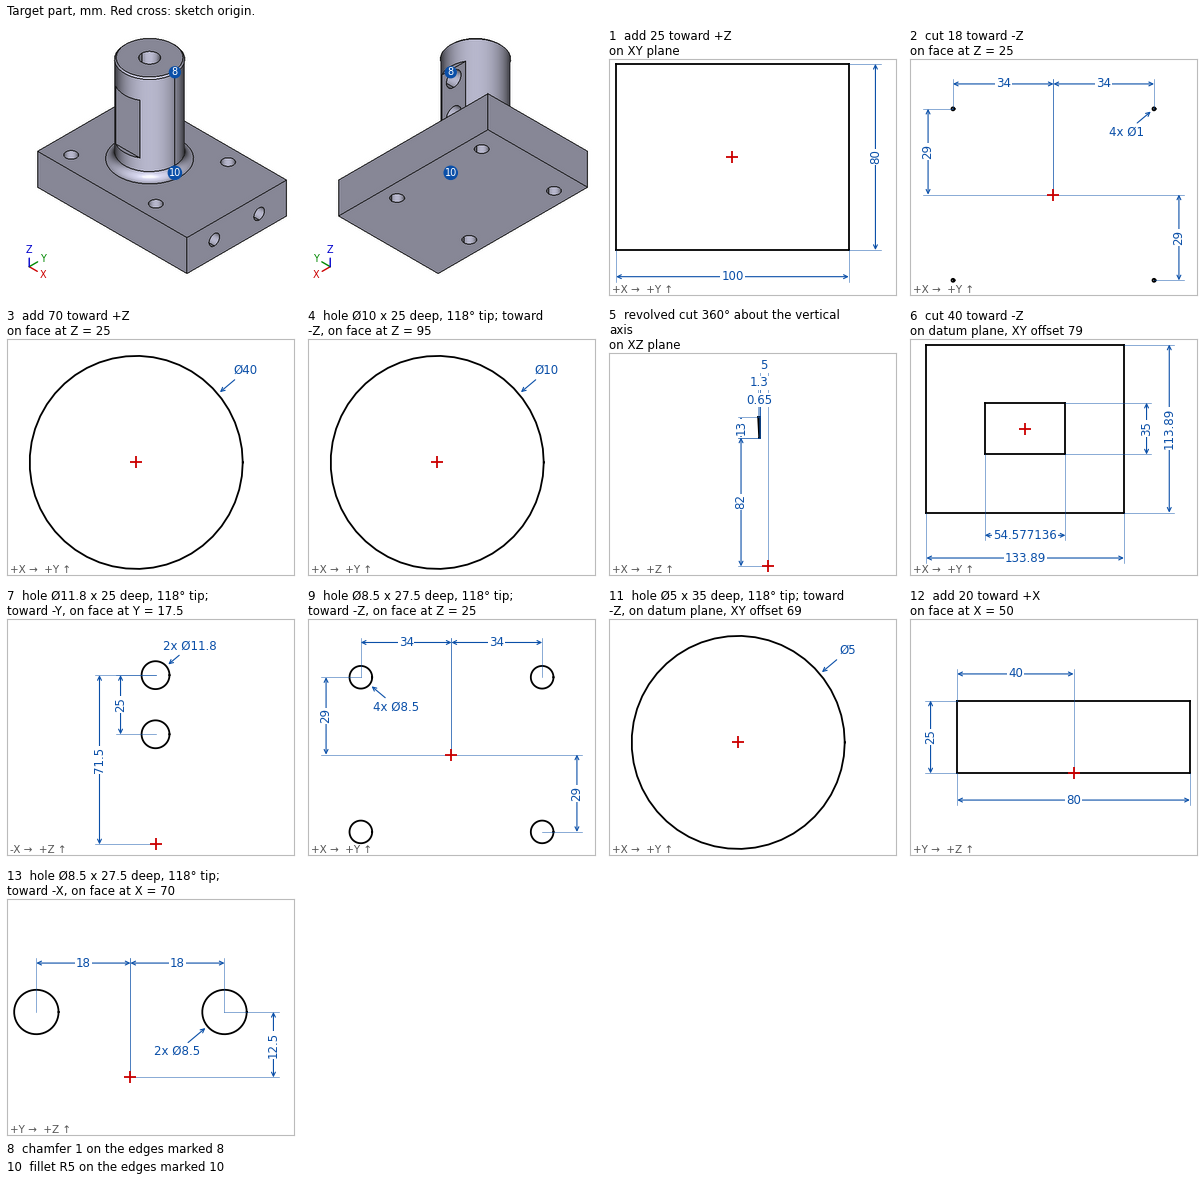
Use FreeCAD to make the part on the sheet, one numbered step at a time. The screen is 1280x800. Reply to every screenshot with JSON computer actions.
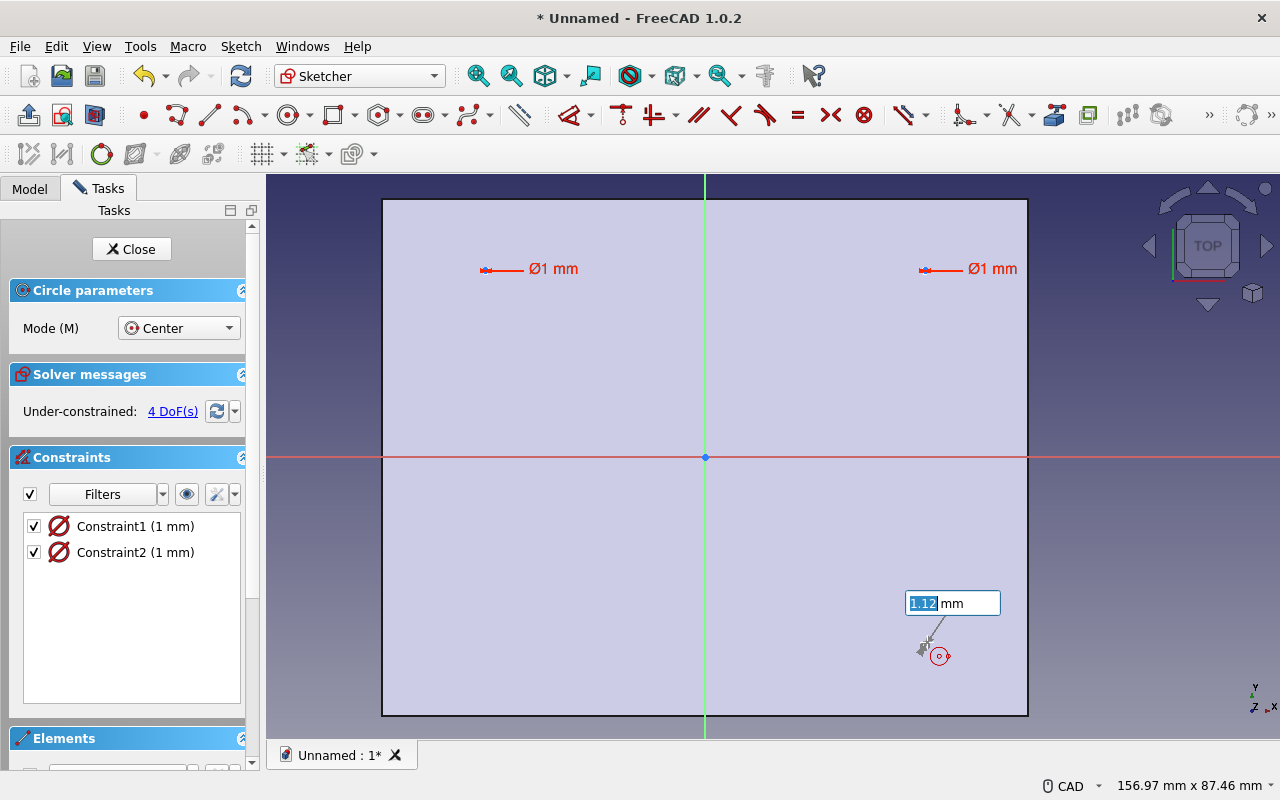
{"action": "type", "text": "1"}
{"action": "key", "text": "Return"}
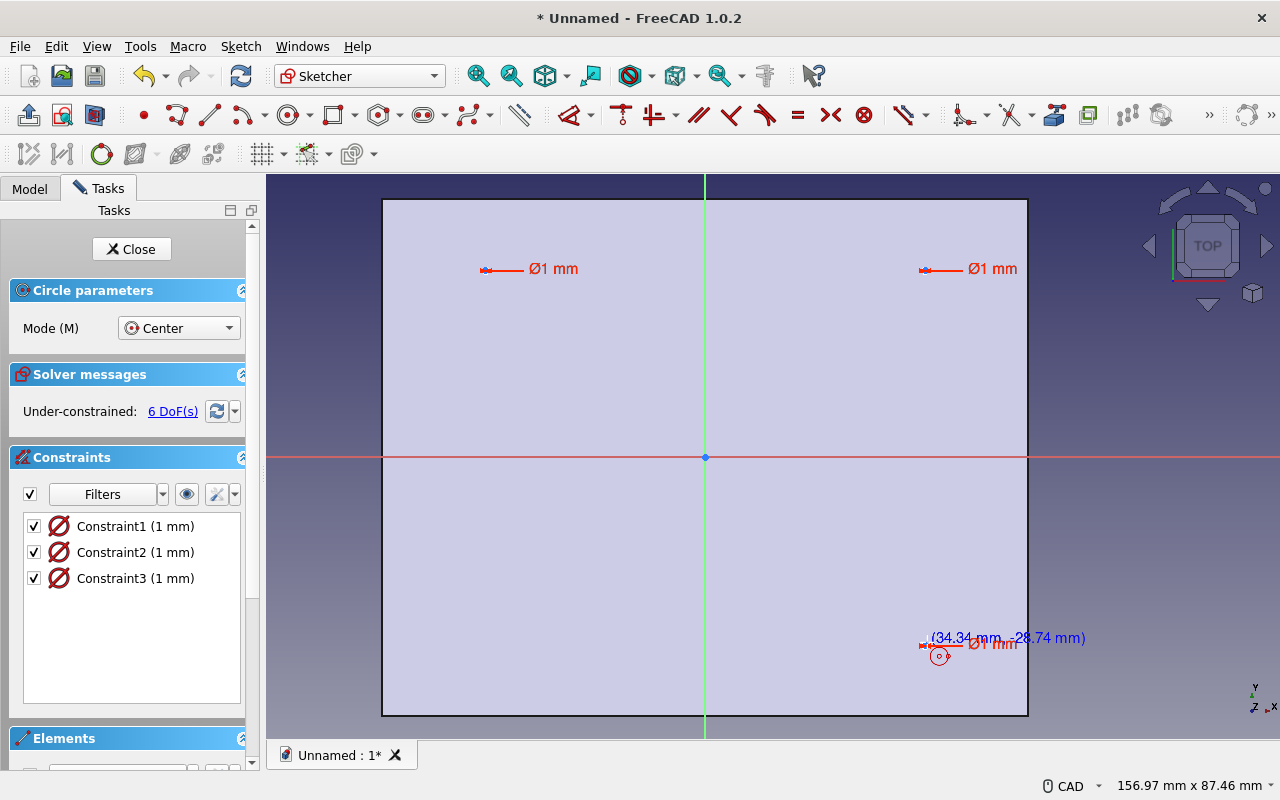
{"action": "scroll", "coordinate": [486, 645], "scroll_direction": "up", "scroll_amount": 10}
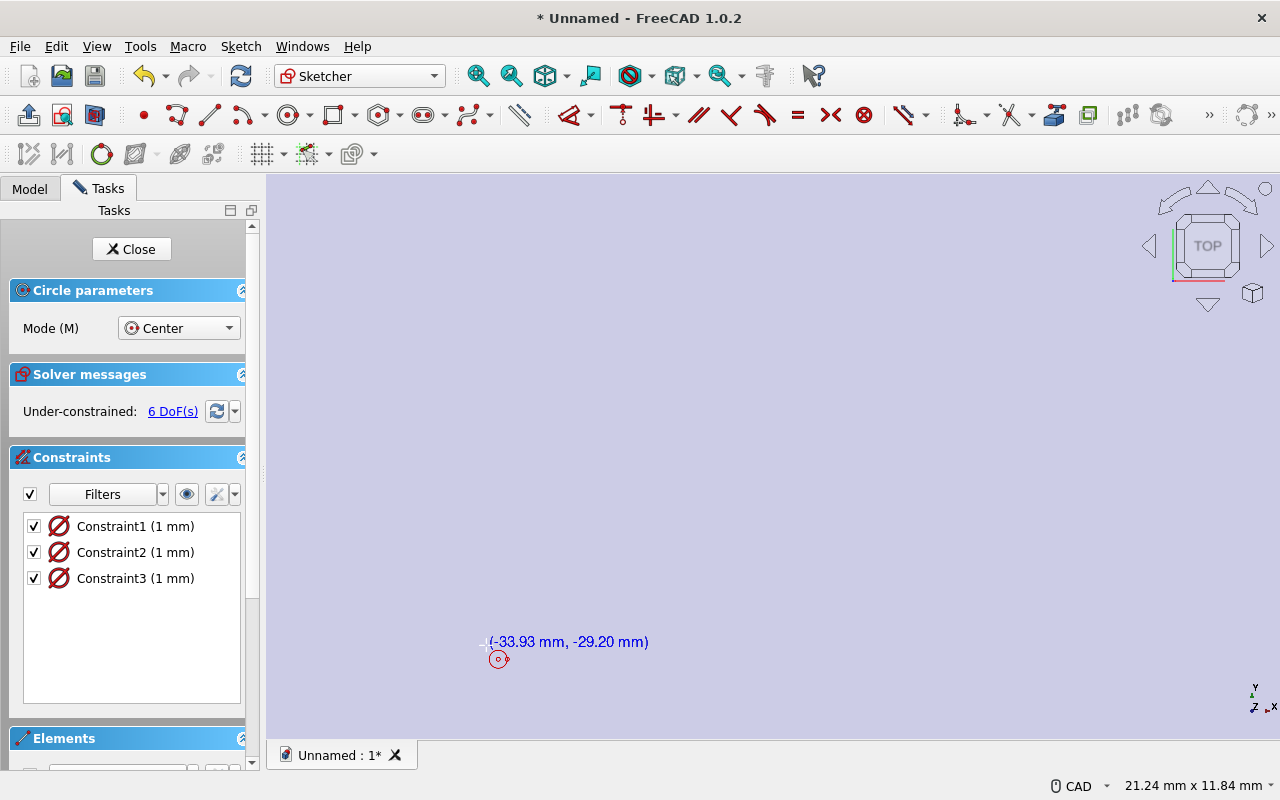
{"action": "scroll", "coordinate": [485, 645], "scroll_direction": "down", "scroll_amount": 10}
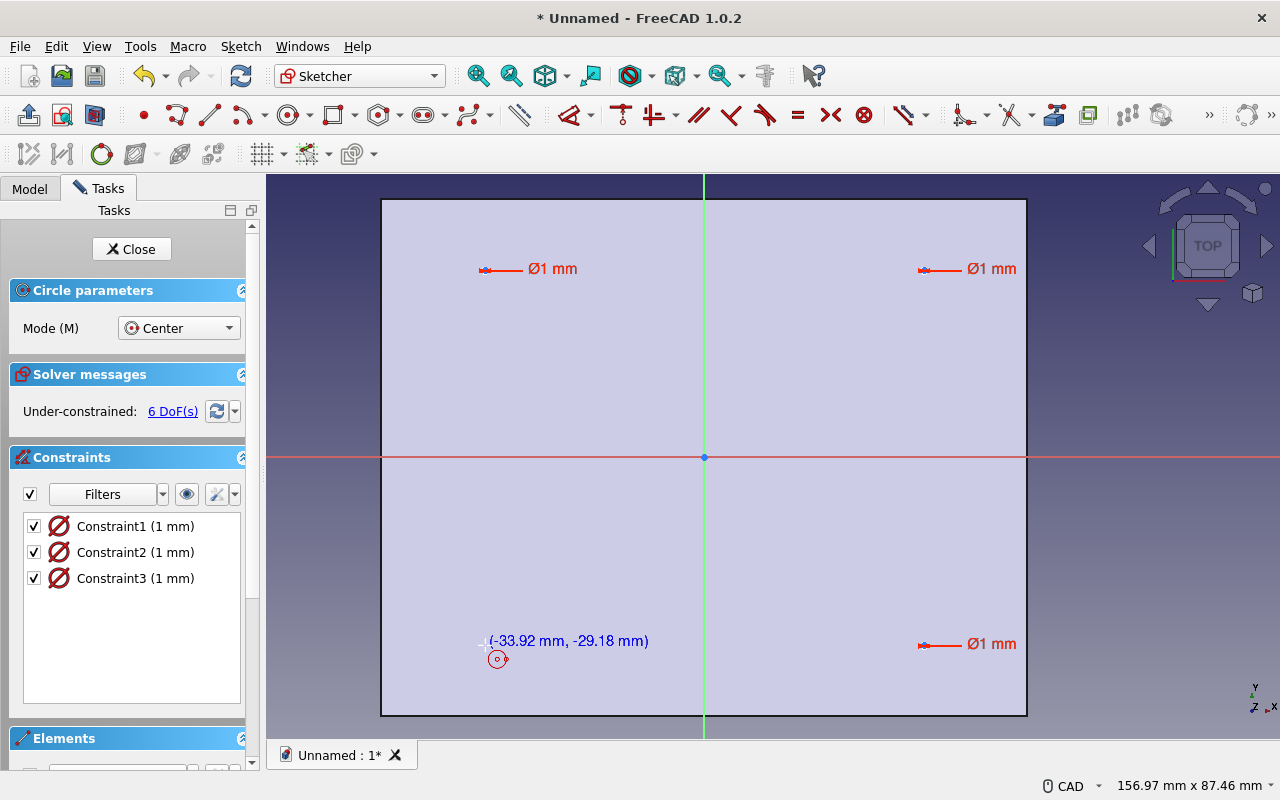
{"action": "left_click", "coordinate": [485, 645]}
{"action": "mouse_move", "coordinate": [487, 642]}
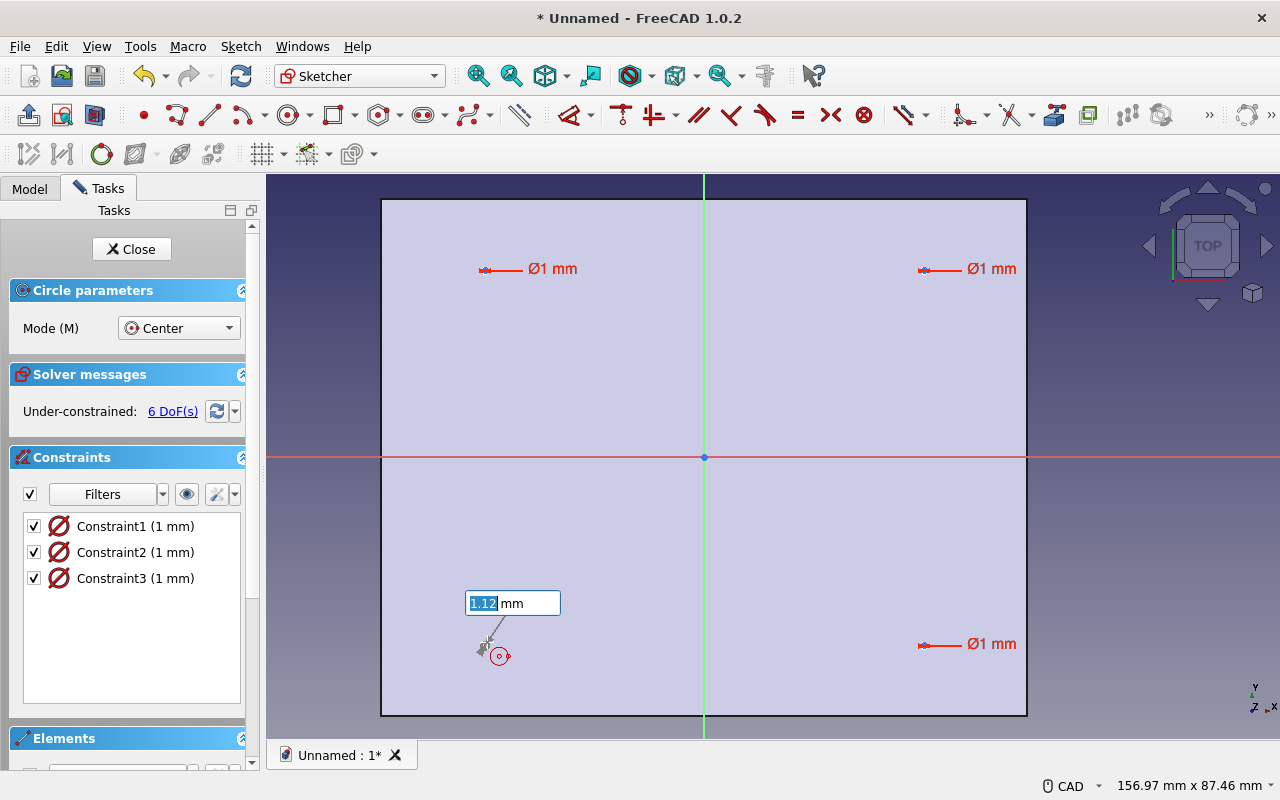
{"action": "type", "text": "1"}
{"action": "key", "text": "Return"}
{"action": "key", "text": "Escape"}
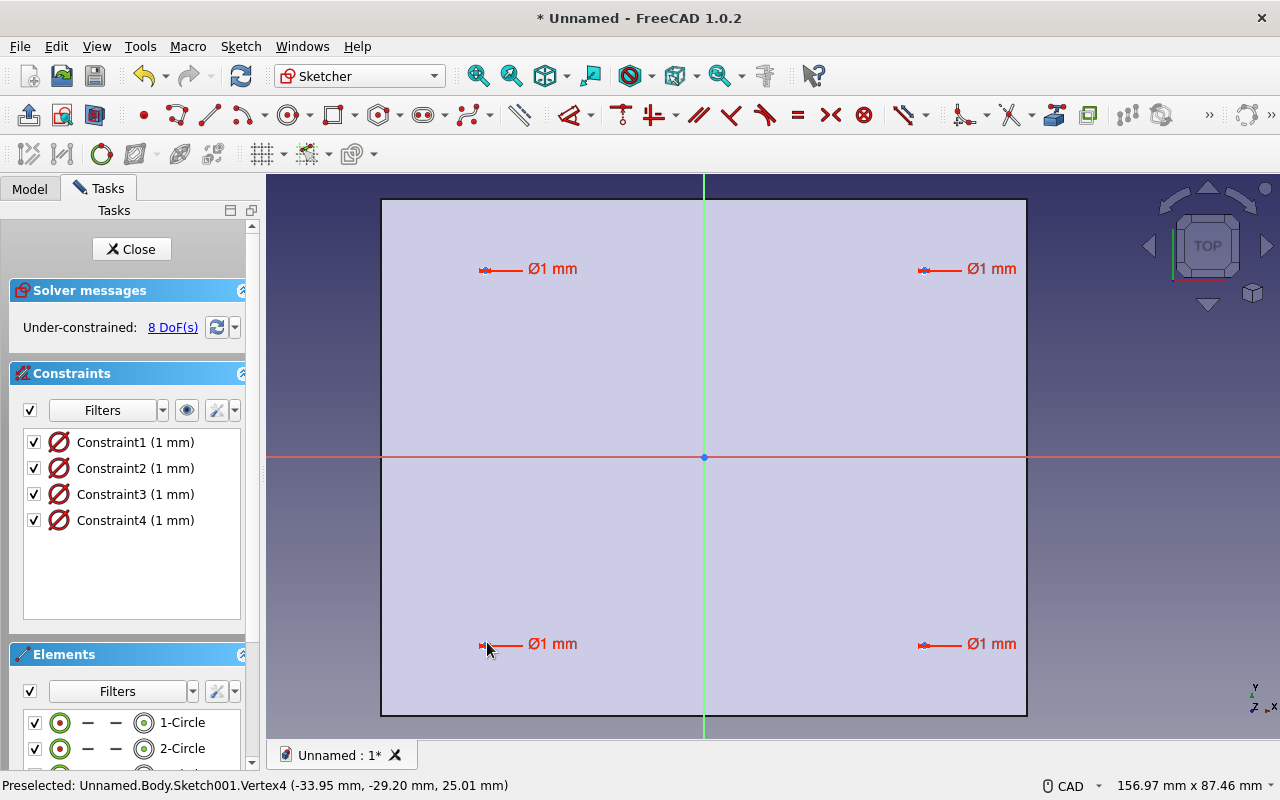
{"action": "left_click", "coordinate": [485, 271]}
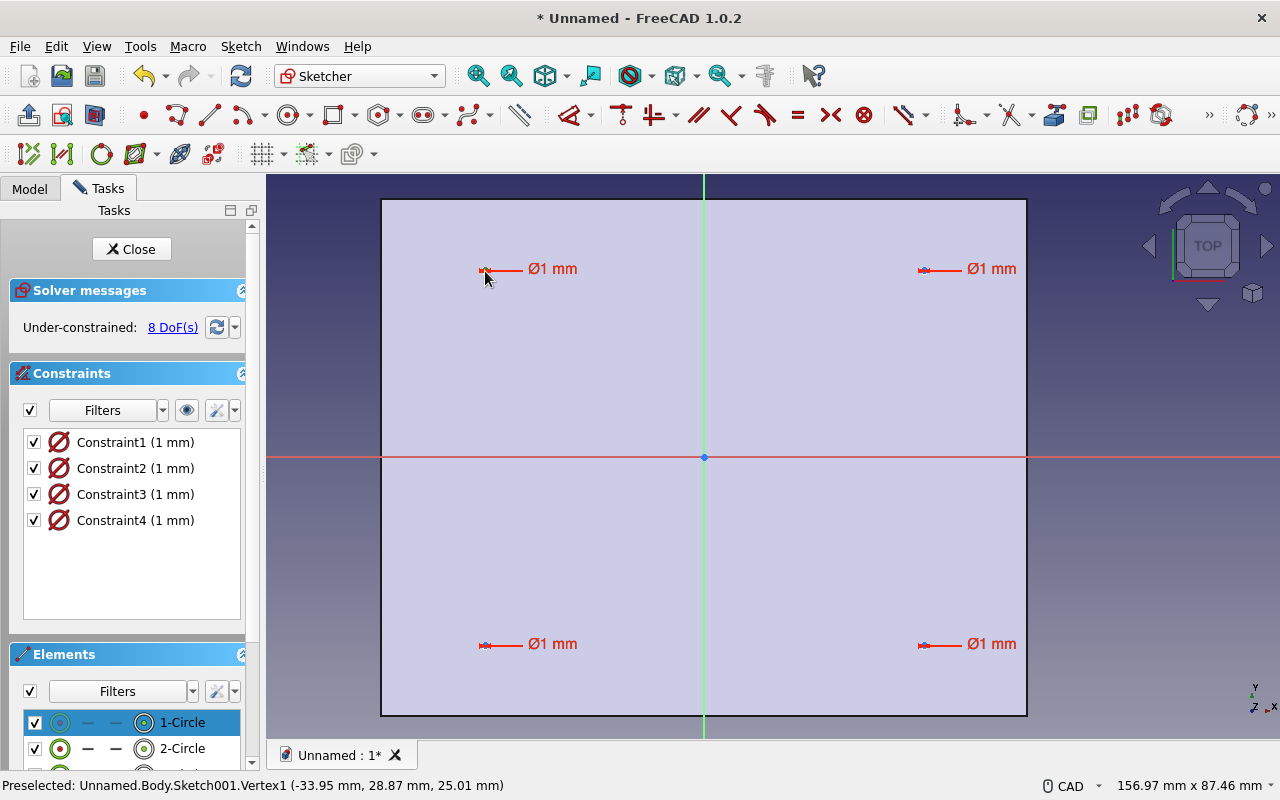
{"action": "left_click", "coordinate": [924, 271]}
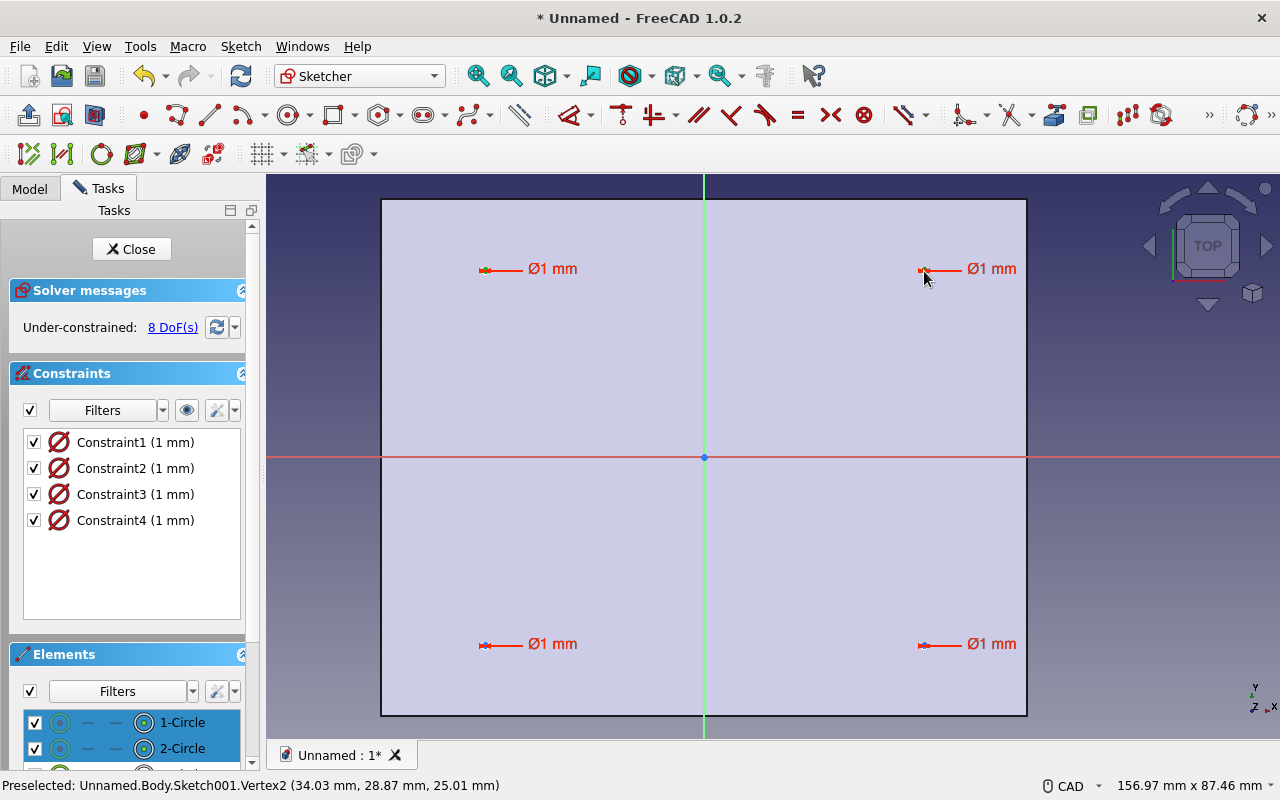
{"action": "key", "text": "h"}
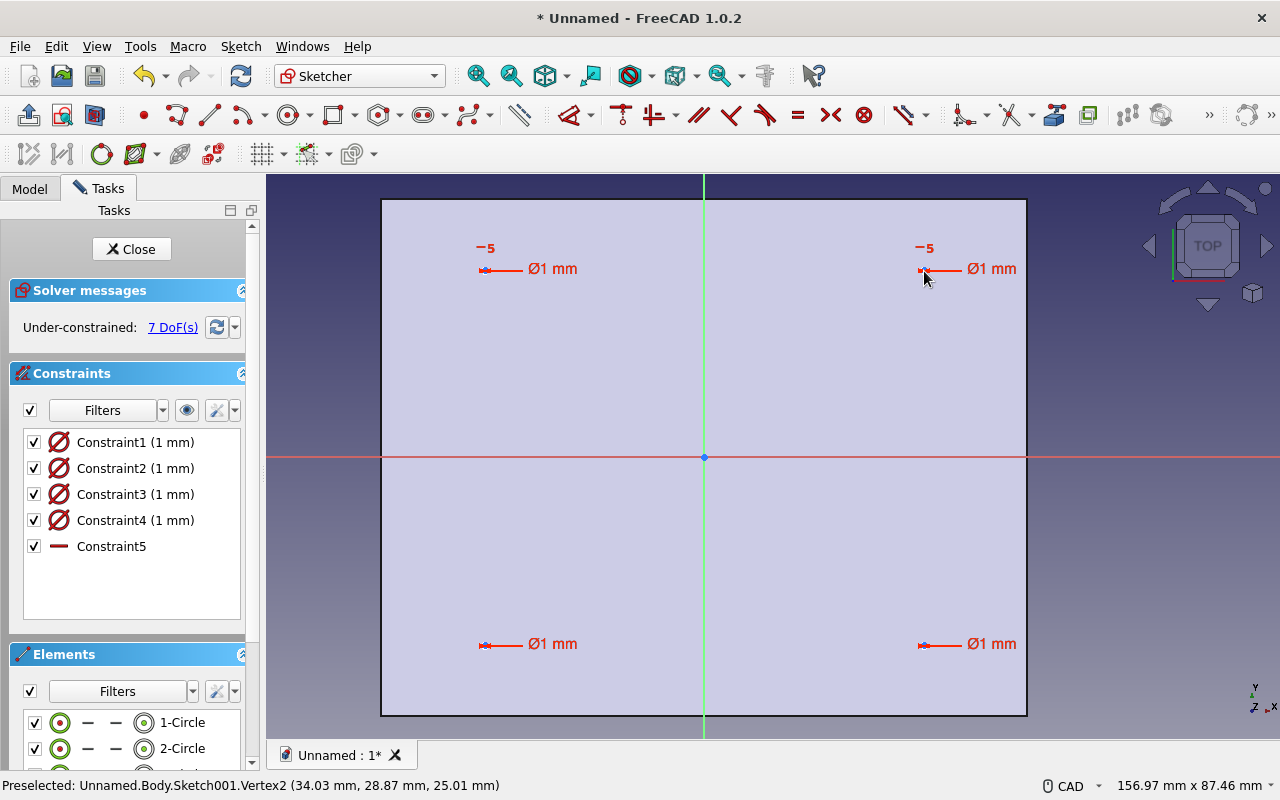
{"action": "left_click", "coordinate": [924, 271]}